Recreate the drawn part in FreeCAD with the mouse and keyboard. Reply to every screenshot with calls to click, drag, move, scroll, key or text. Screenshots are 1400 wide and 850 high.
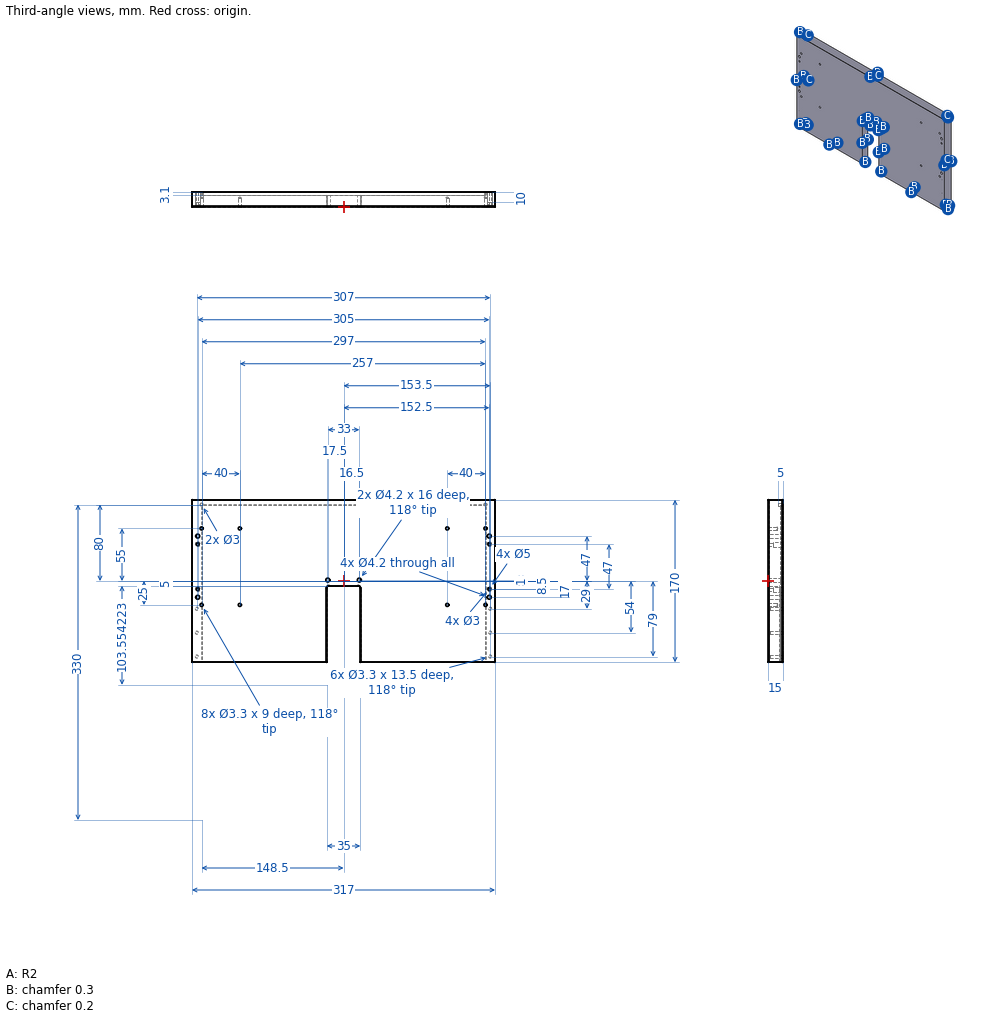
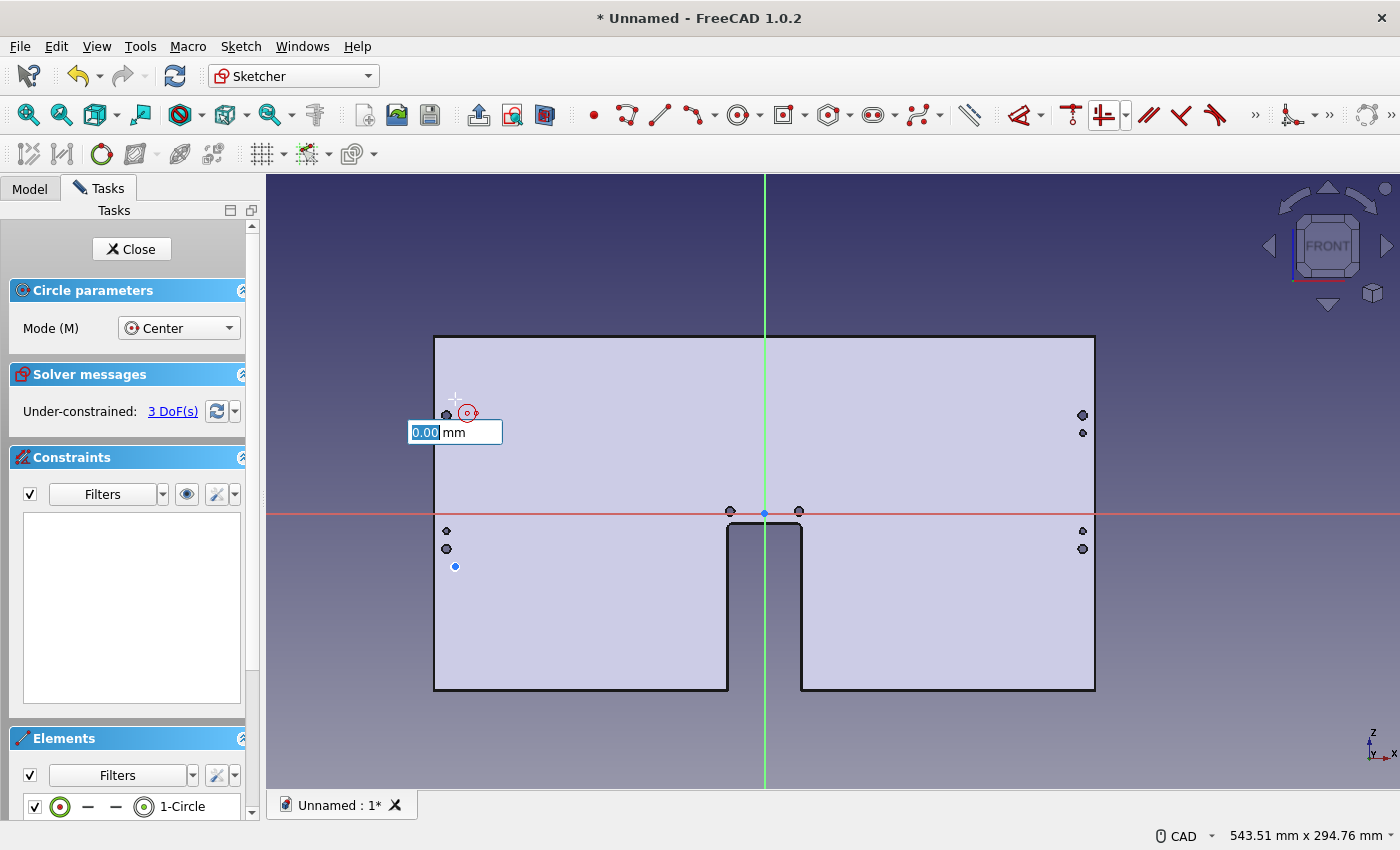
scroll(457, 396, up, 8)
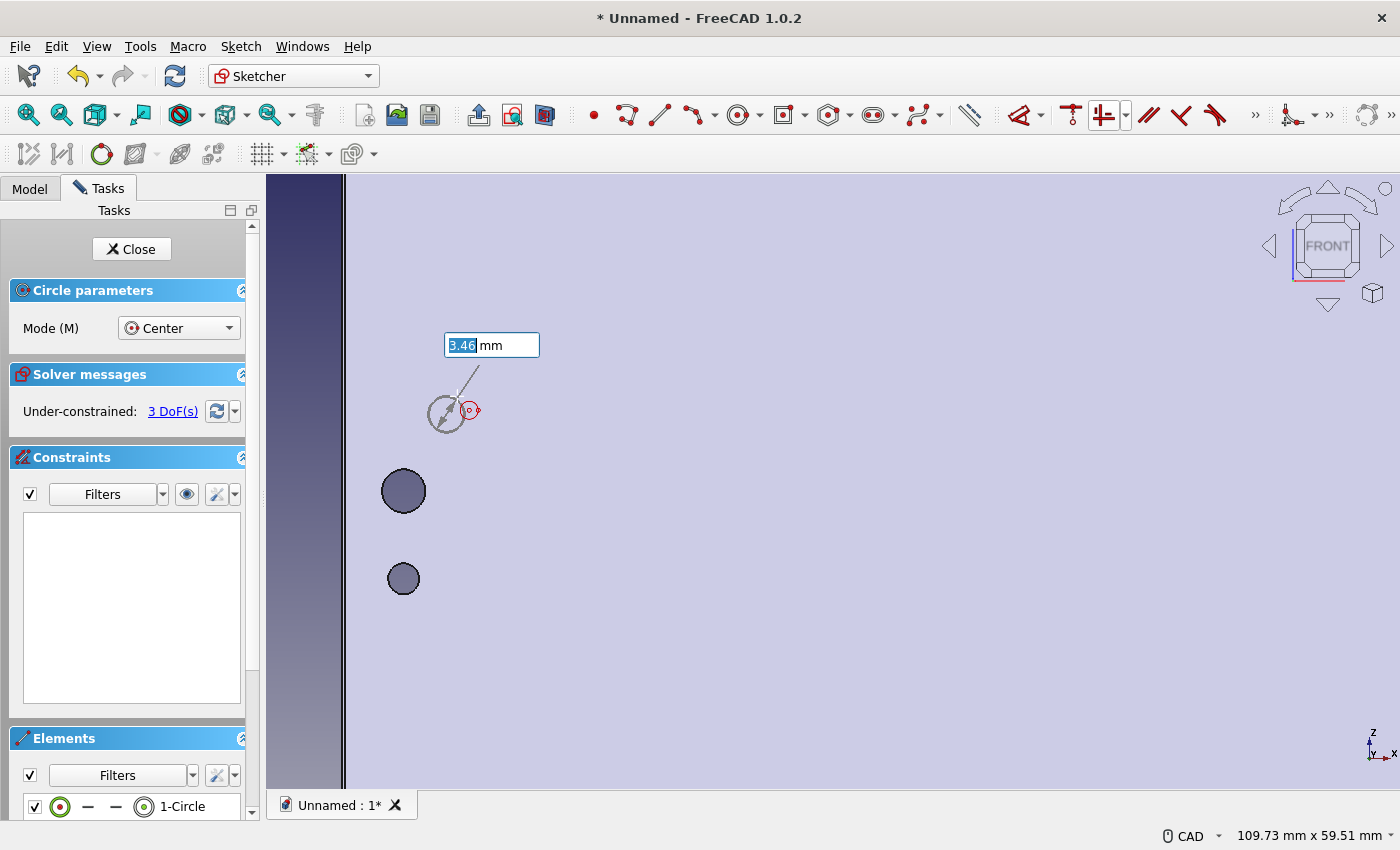
click(457, 396)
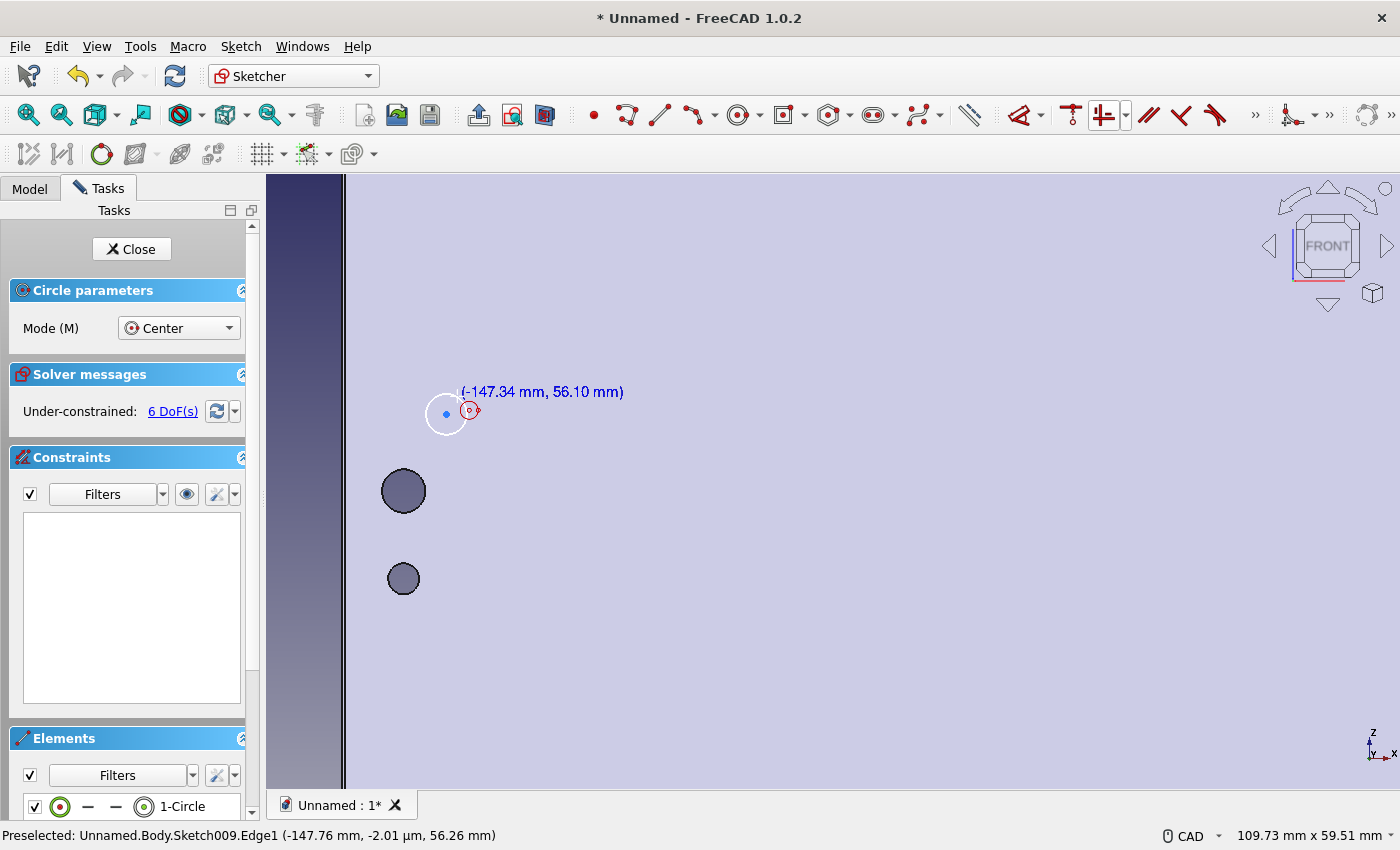
scroll(457, 395, down, 8)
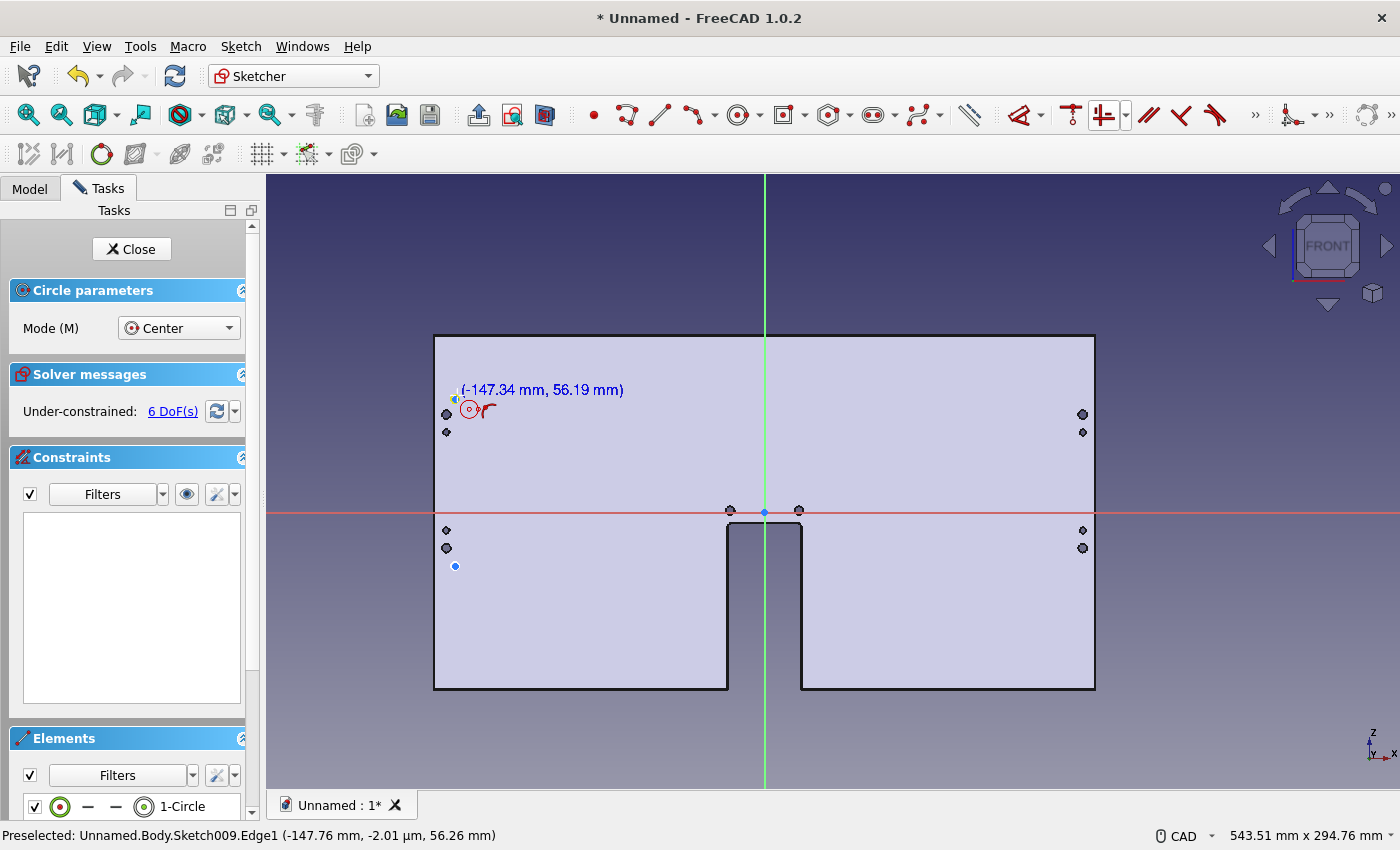
scroll(538, 565, up, 10)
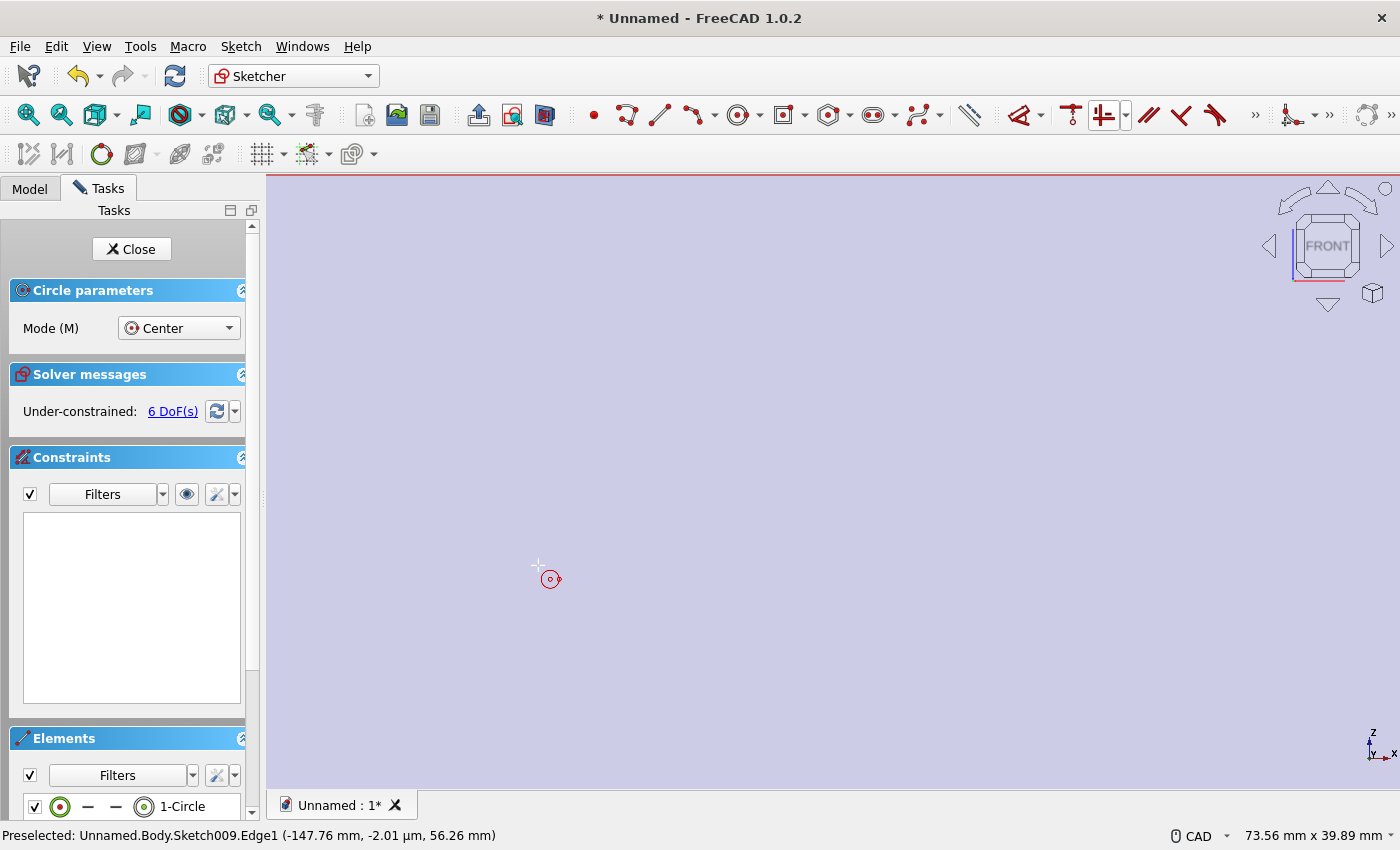
scroll(538, 566, down, 10)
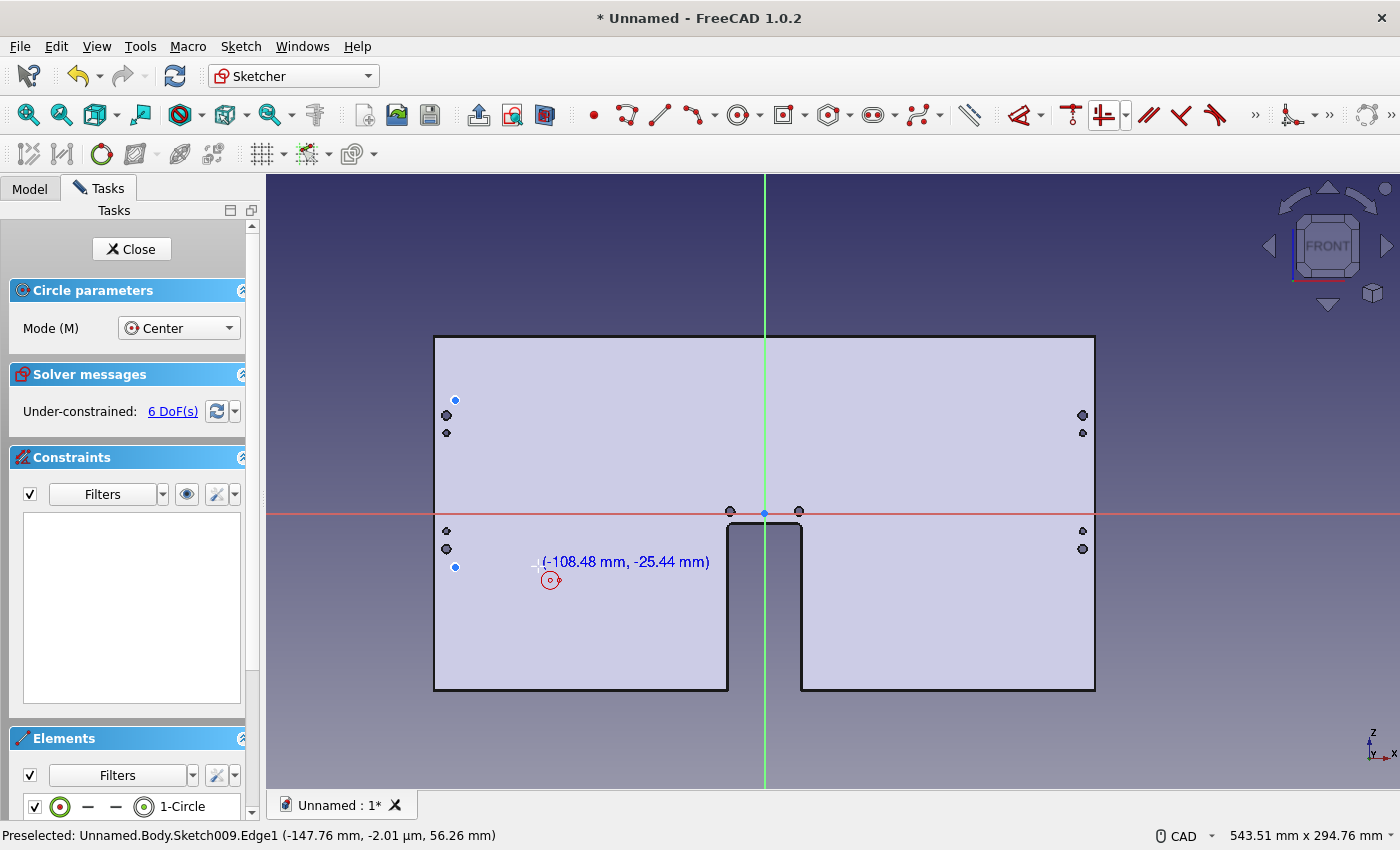
click(538, 566)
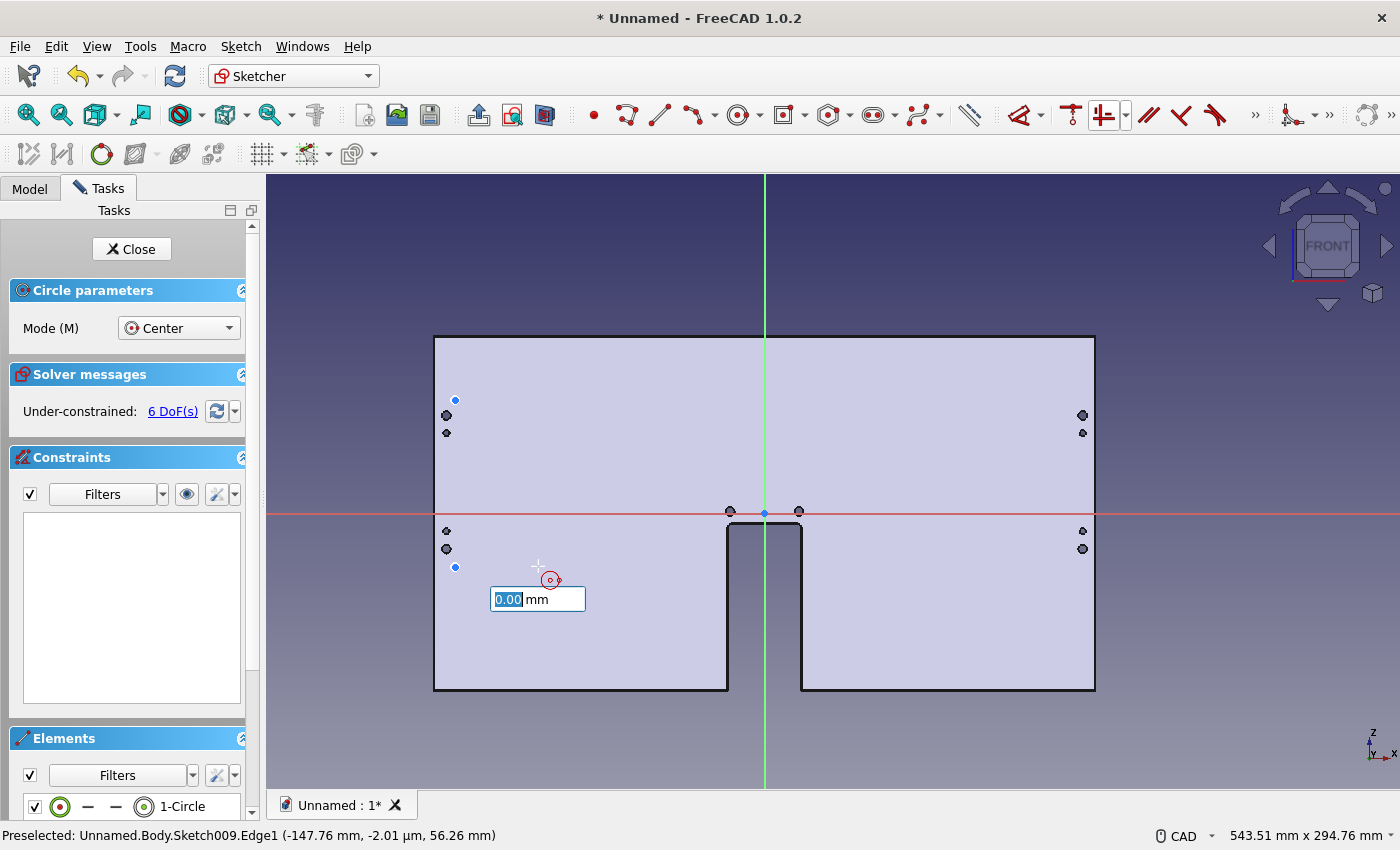
scroll(541, 563, up, 8)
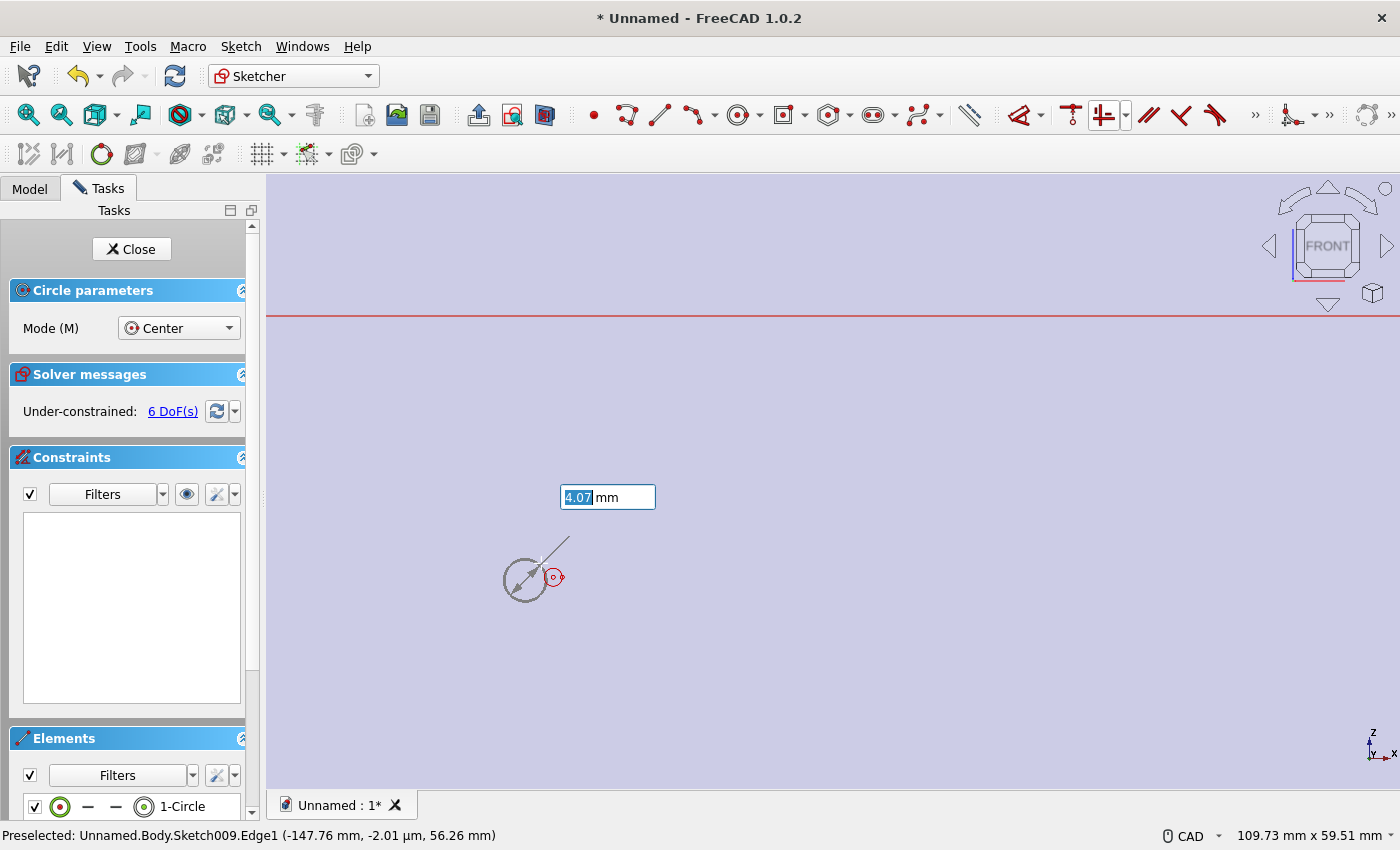
click(538, 562)